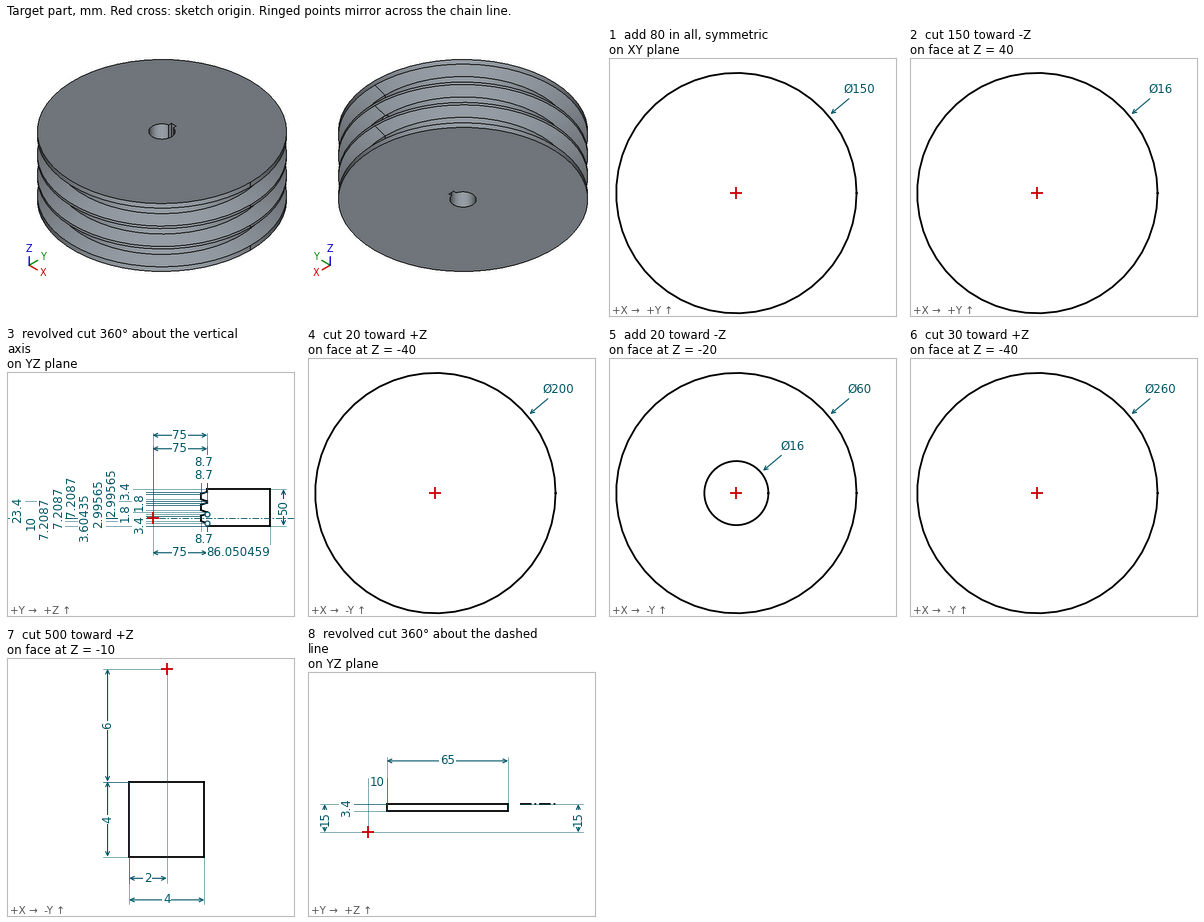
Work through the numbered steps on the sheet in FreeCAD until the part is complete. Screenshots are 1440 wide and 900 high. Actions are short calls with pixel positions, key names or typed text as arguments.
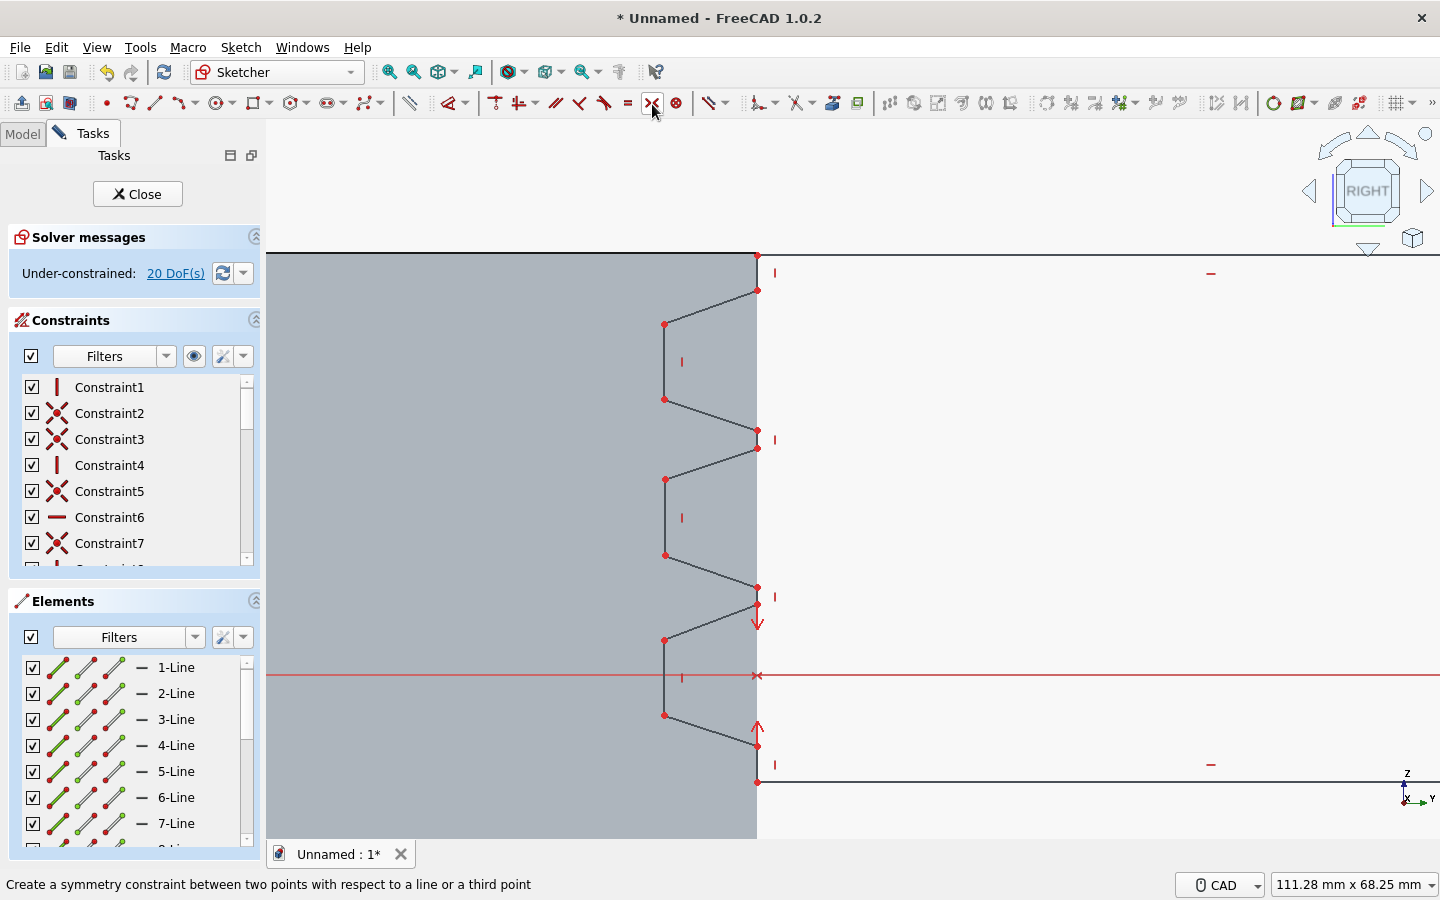
key(d)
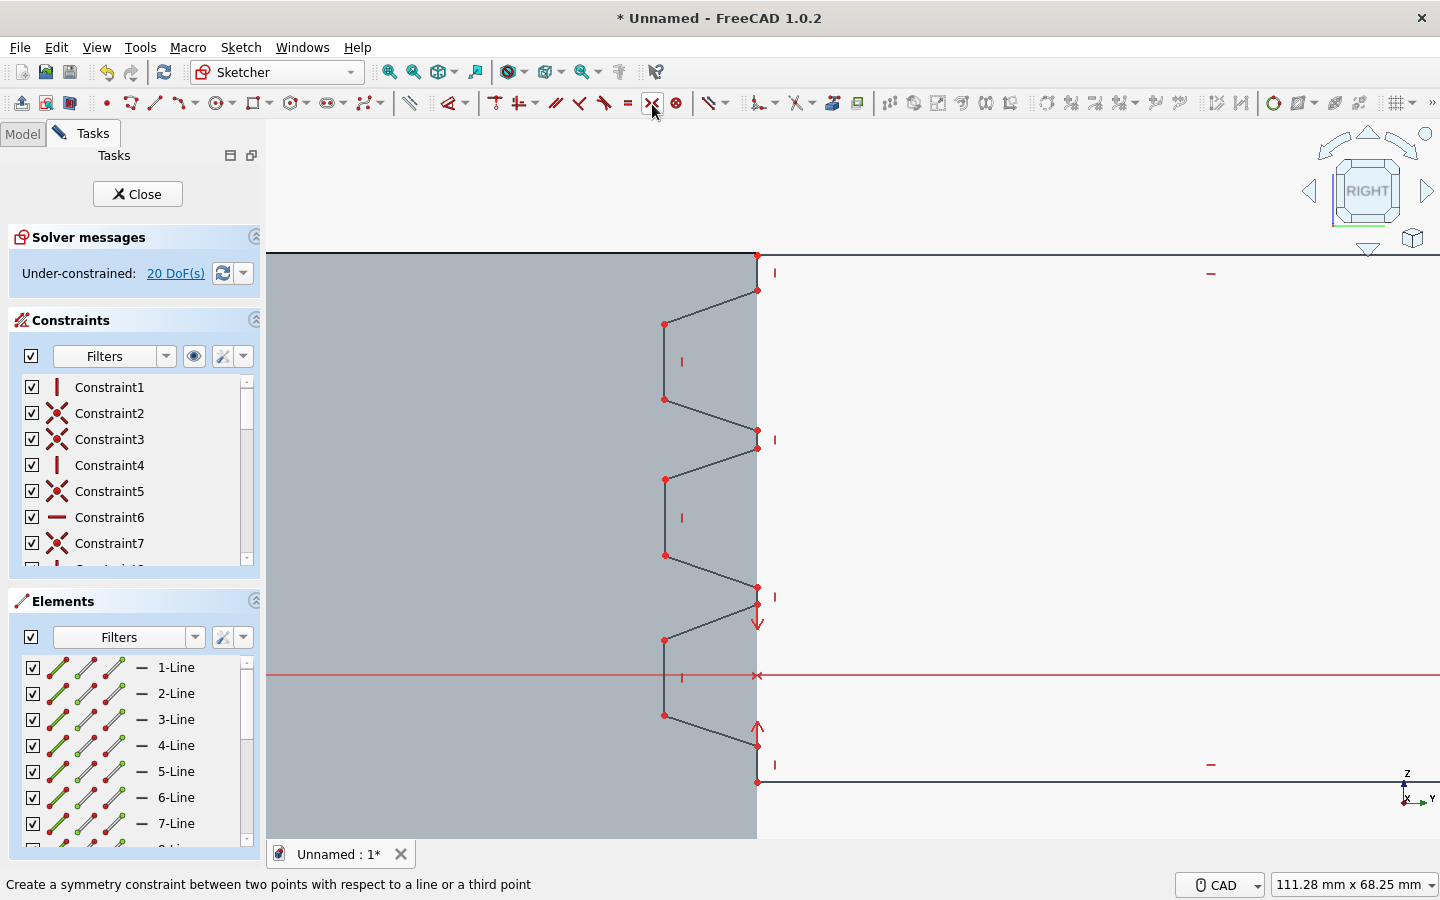
scroll(760, 448, down, 4)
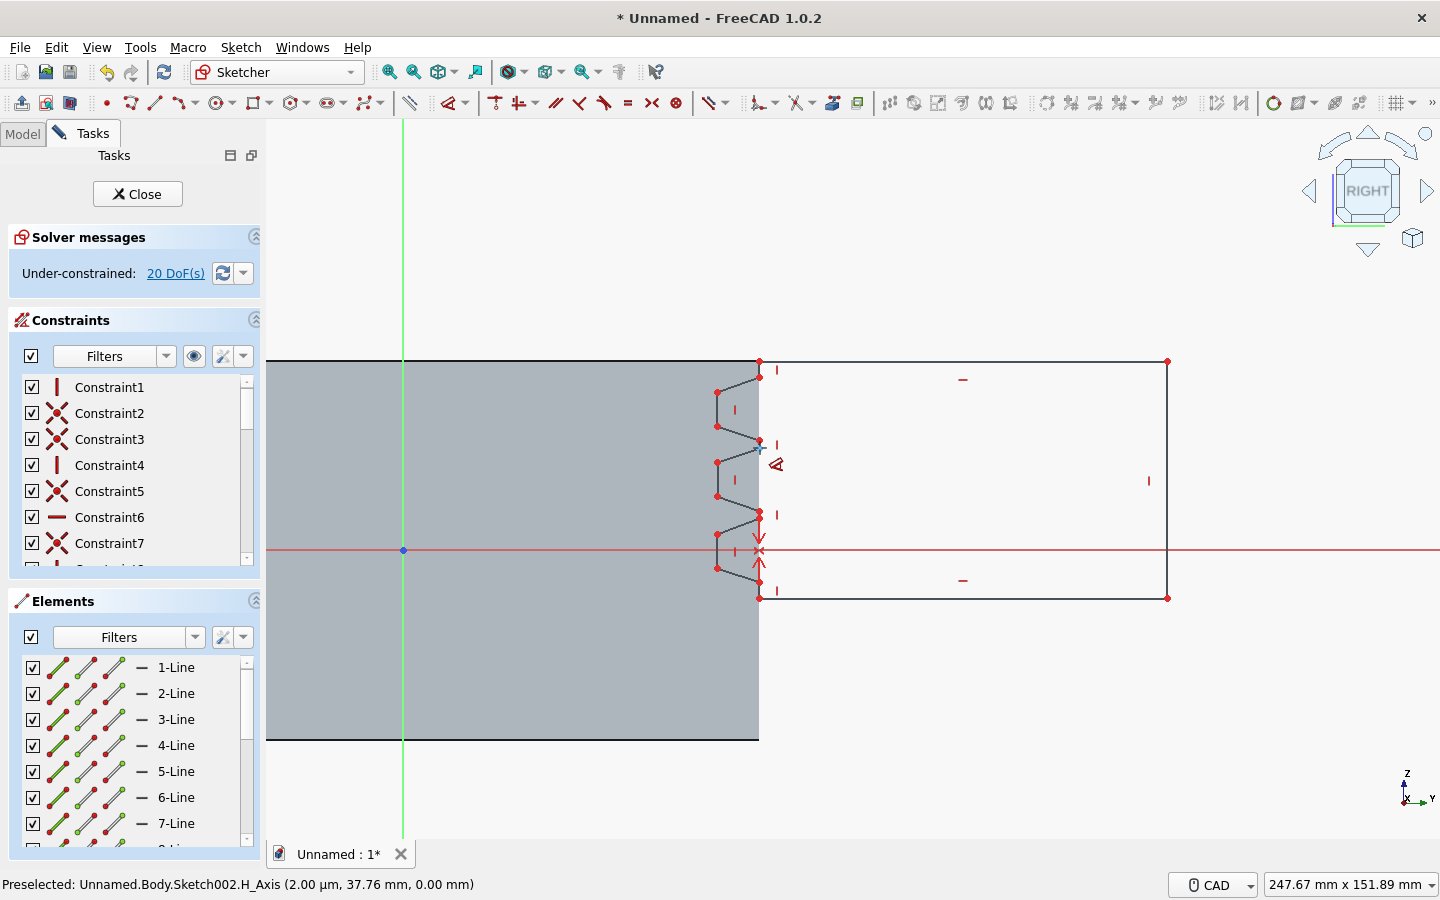
click(1167, 527)
click(1201, 480)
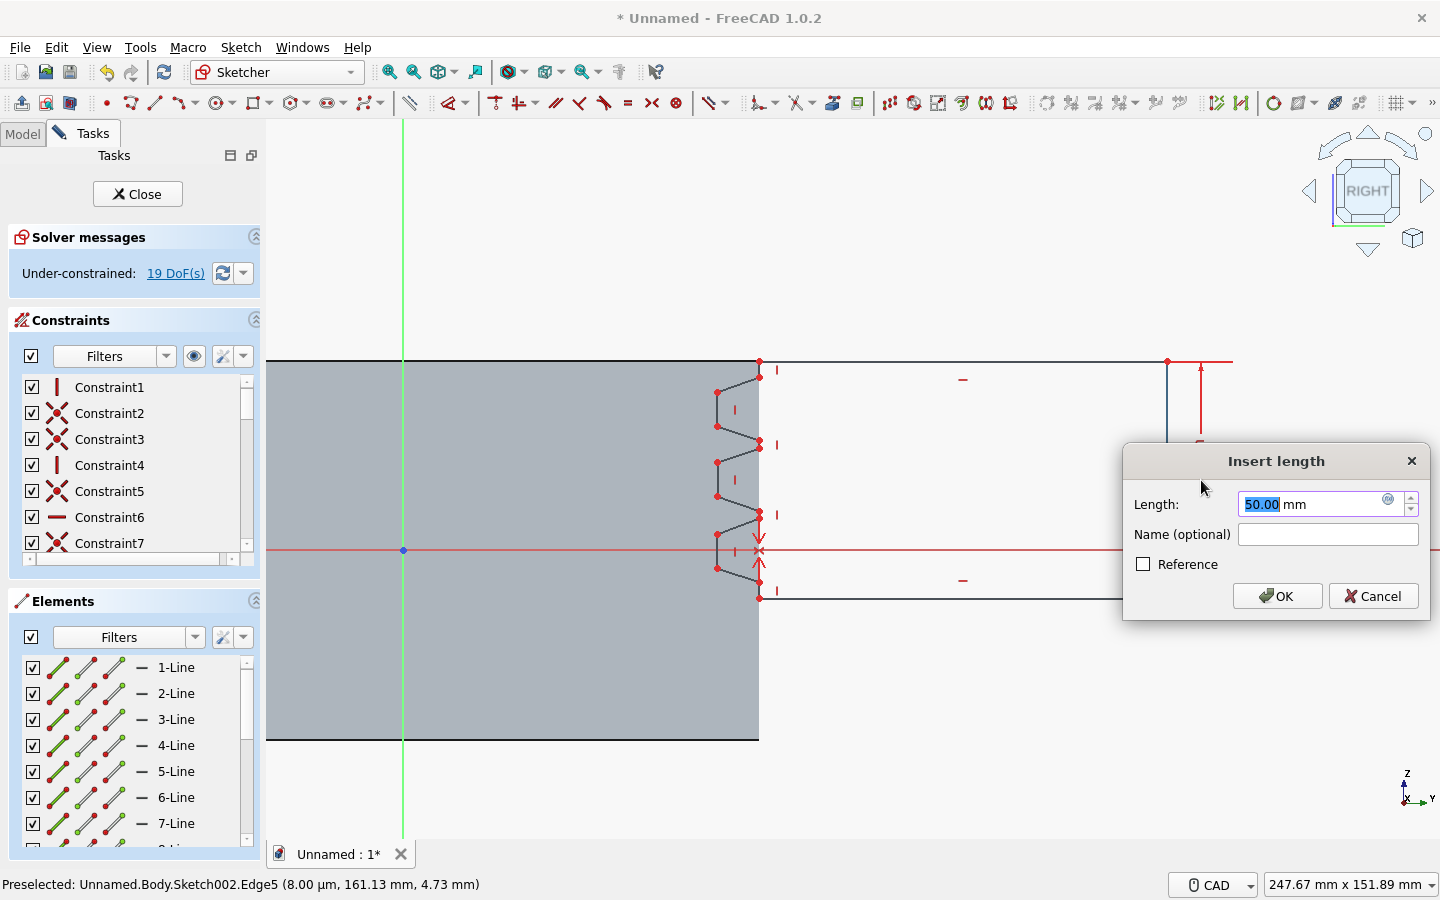
text(50)
key(Return)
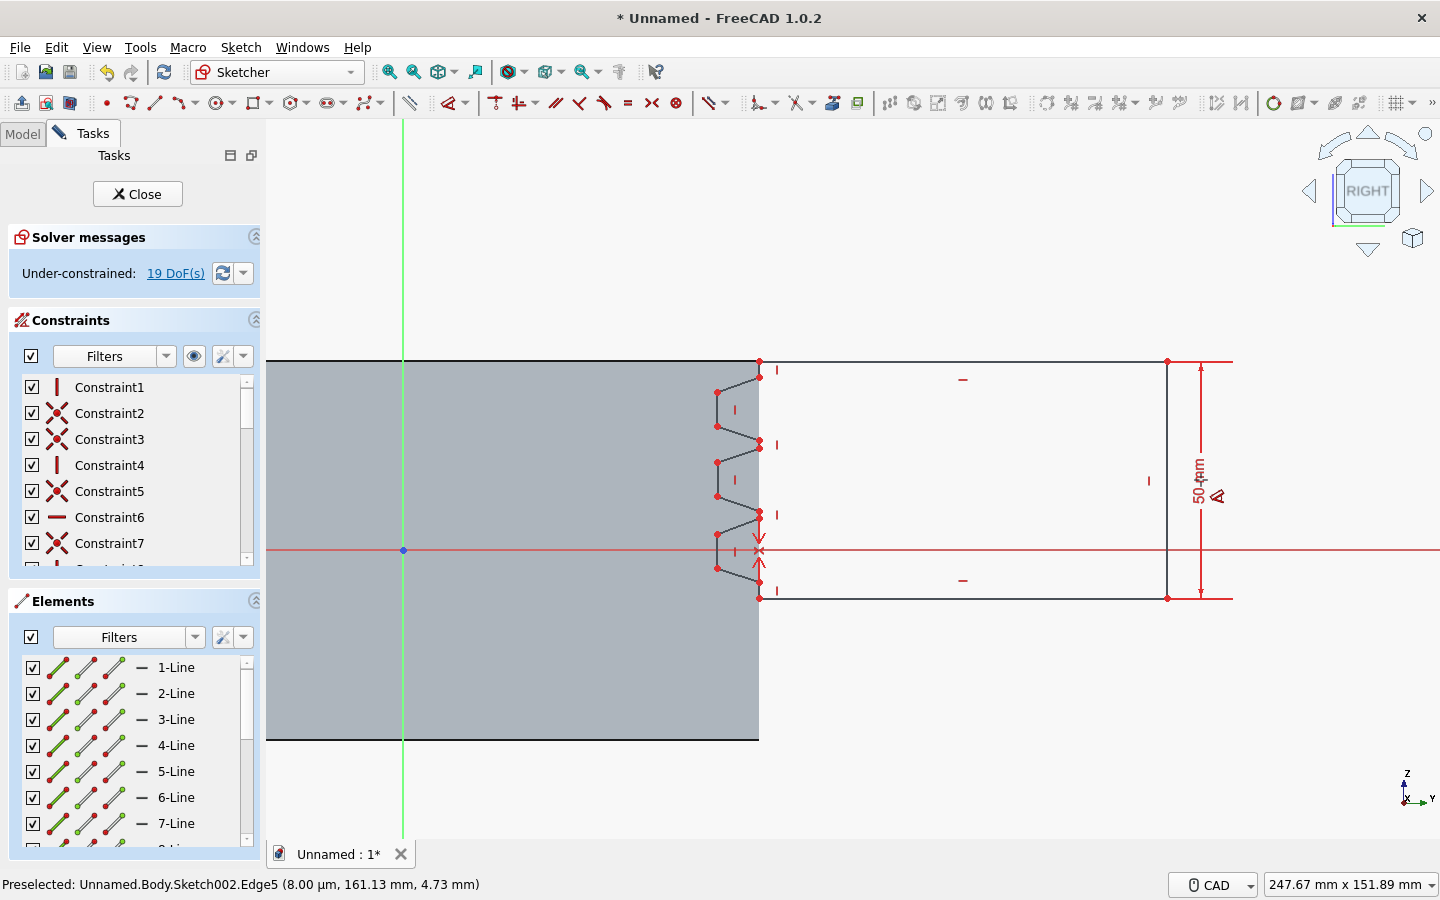
scroll(759, 590, up, 5)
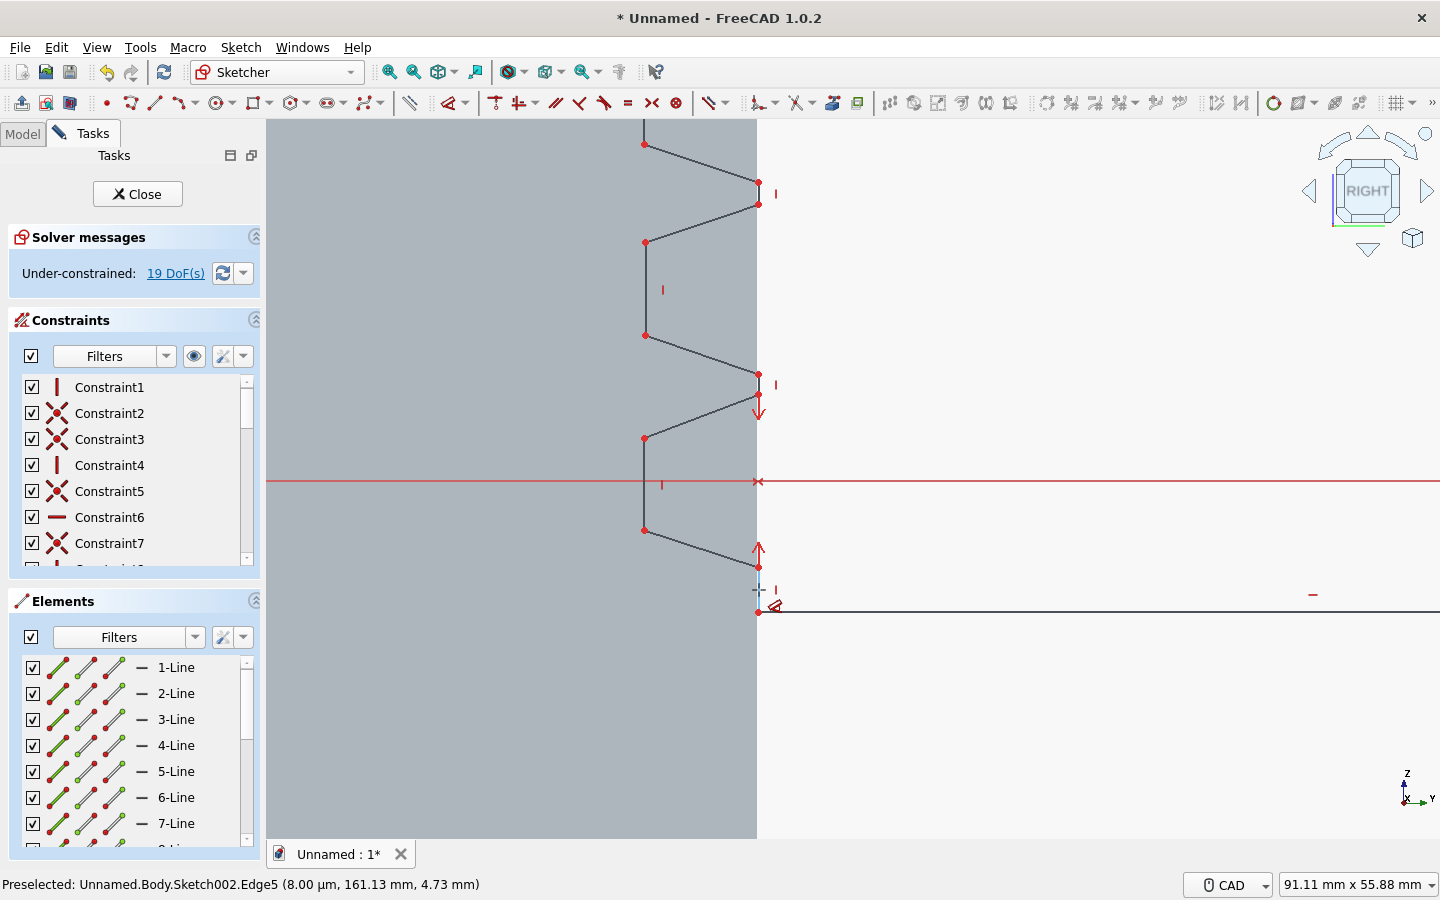
click(759, 590)
click(725, 590)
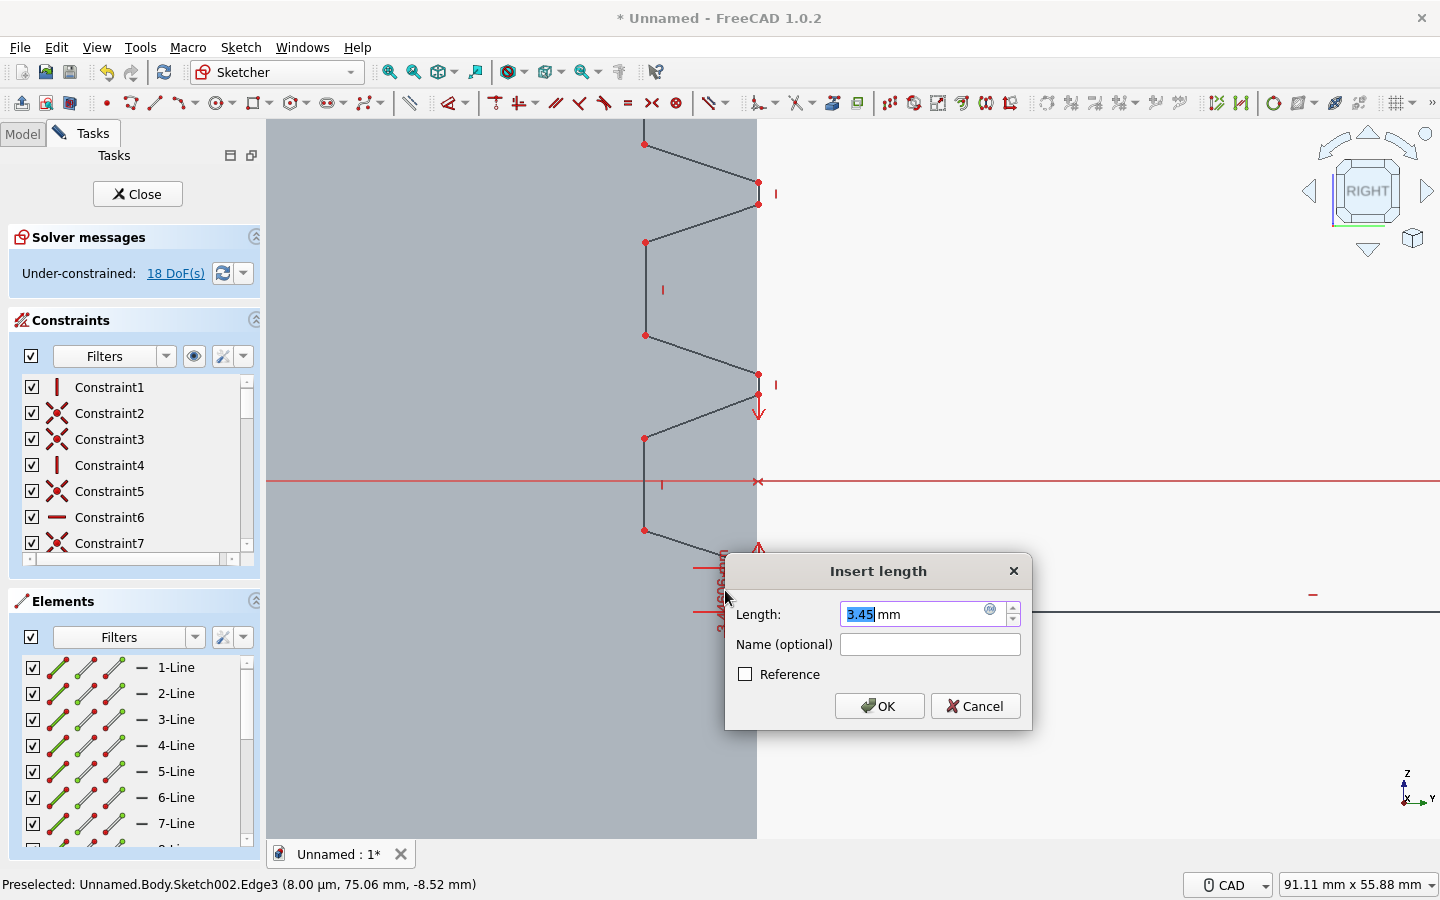
text(3.4)
key(Return)